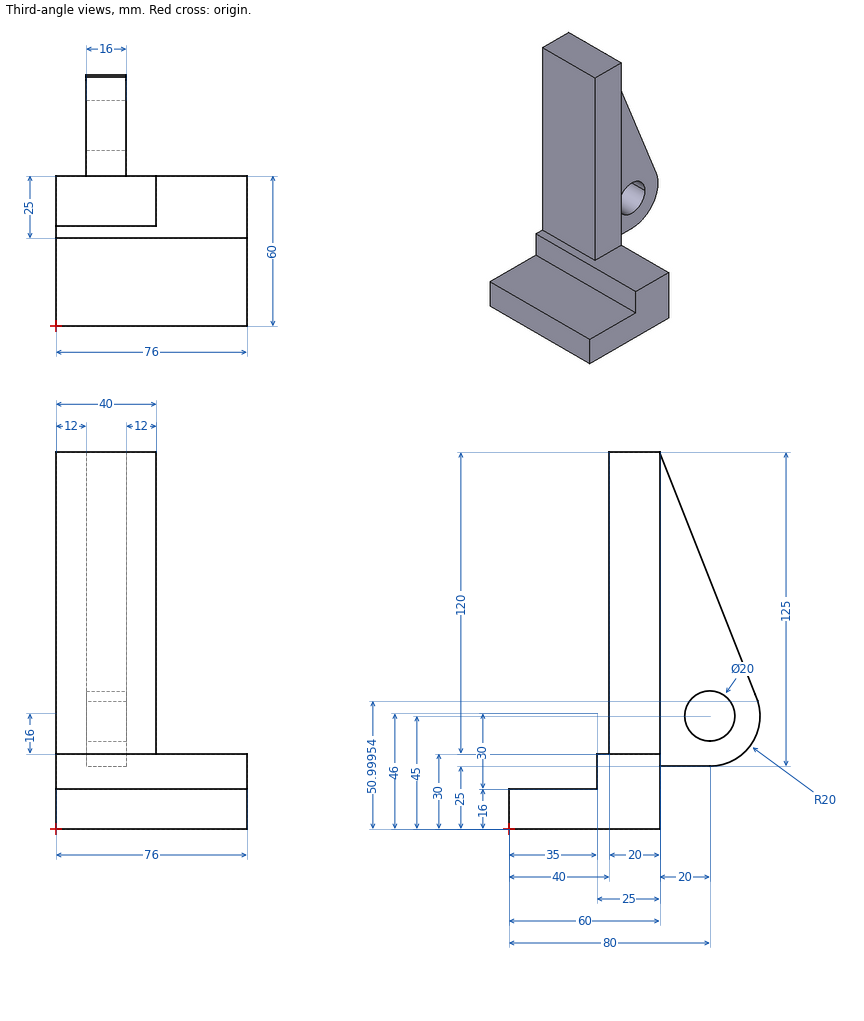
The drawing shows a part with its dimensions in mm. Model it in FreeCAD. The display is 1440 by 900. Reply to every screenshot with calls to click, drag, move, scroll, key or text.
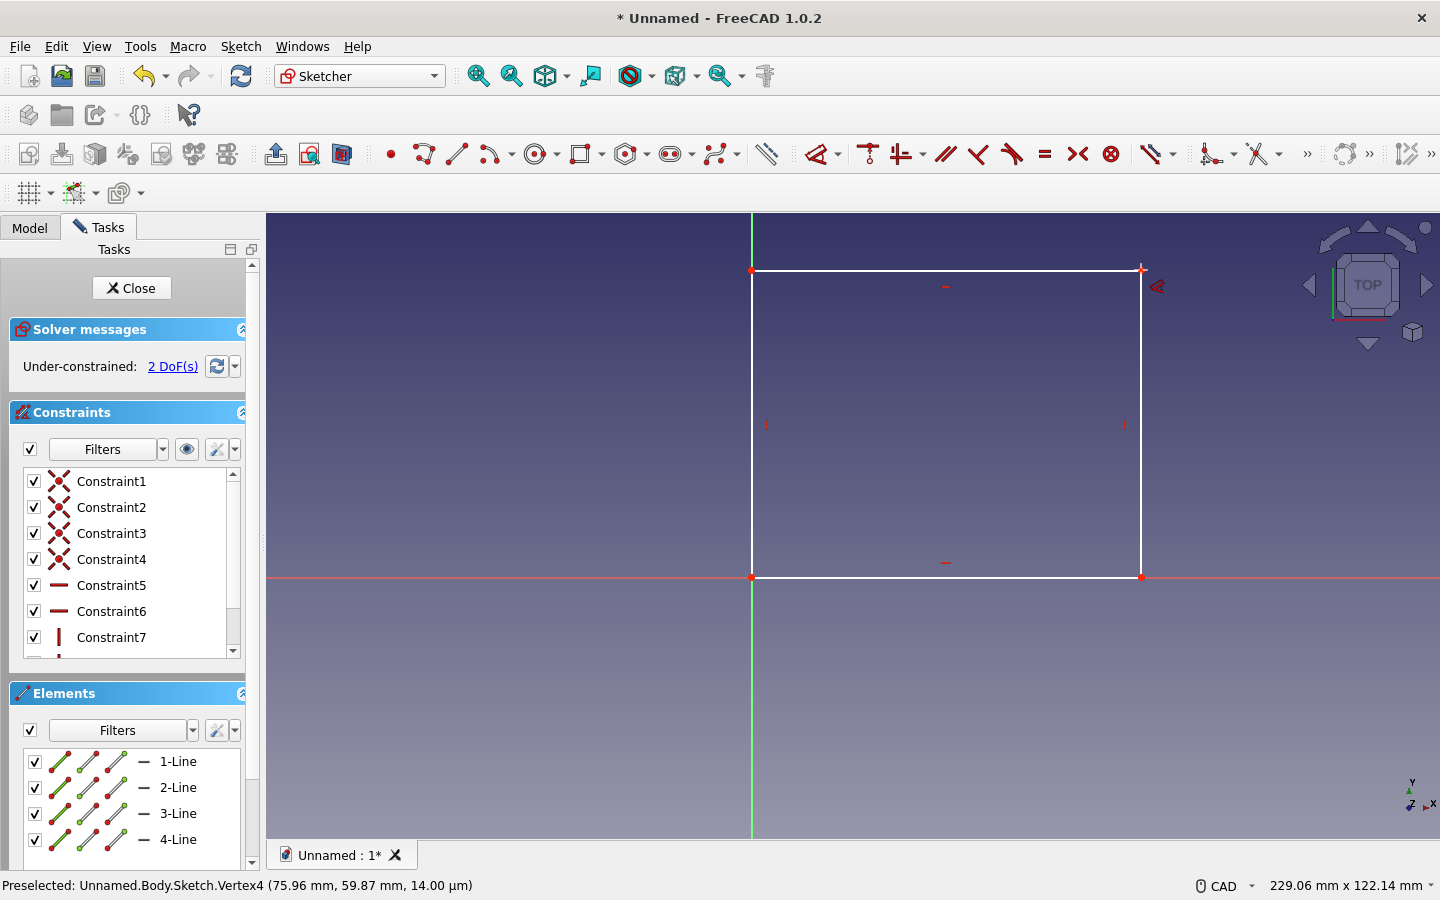
click(868, 578)
click(946, 612)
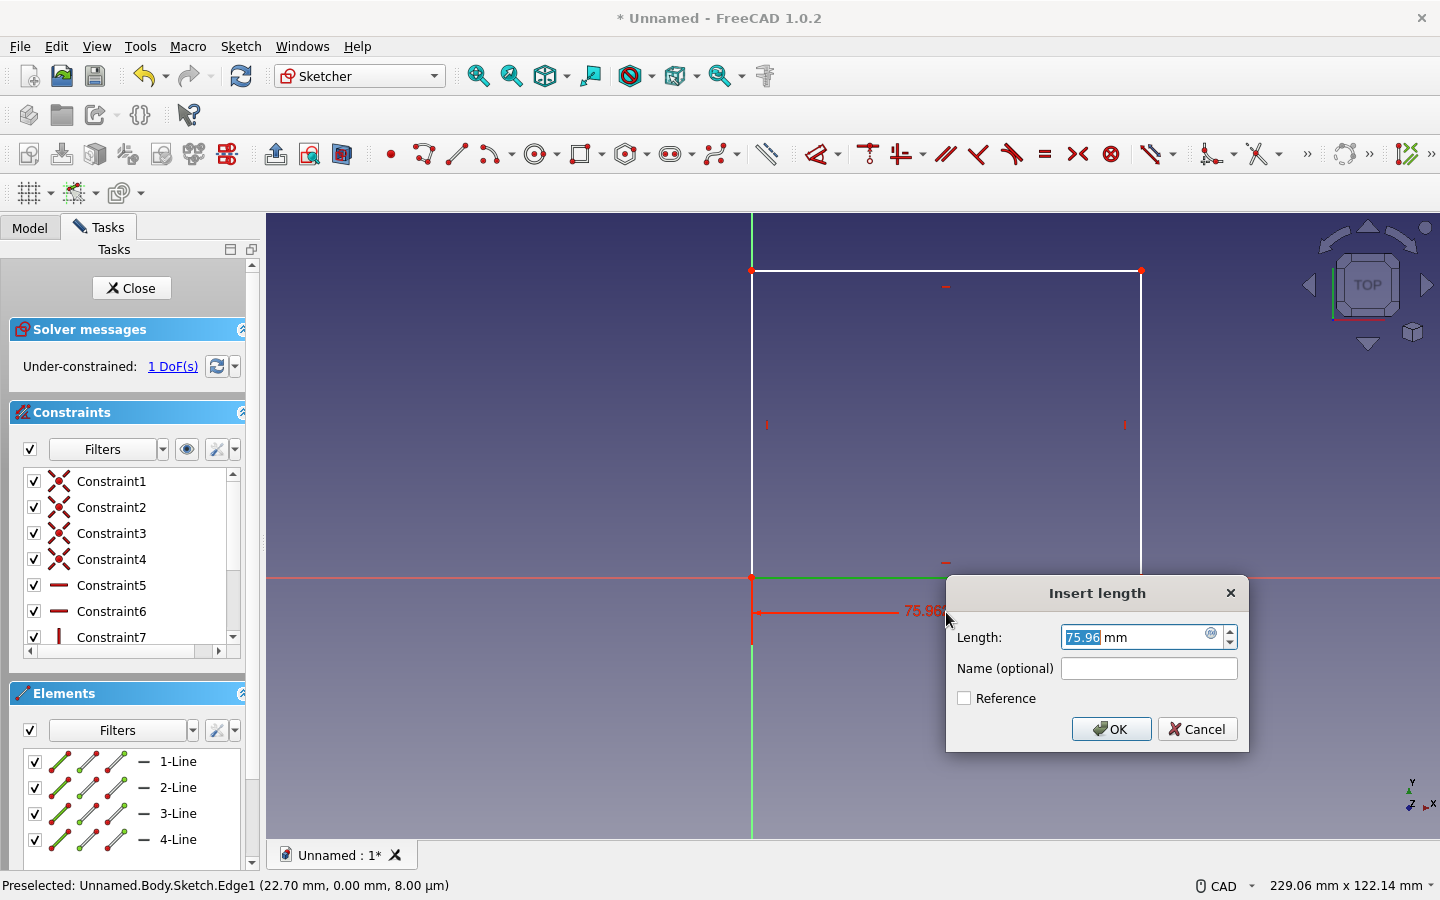
text(76)
key(Return)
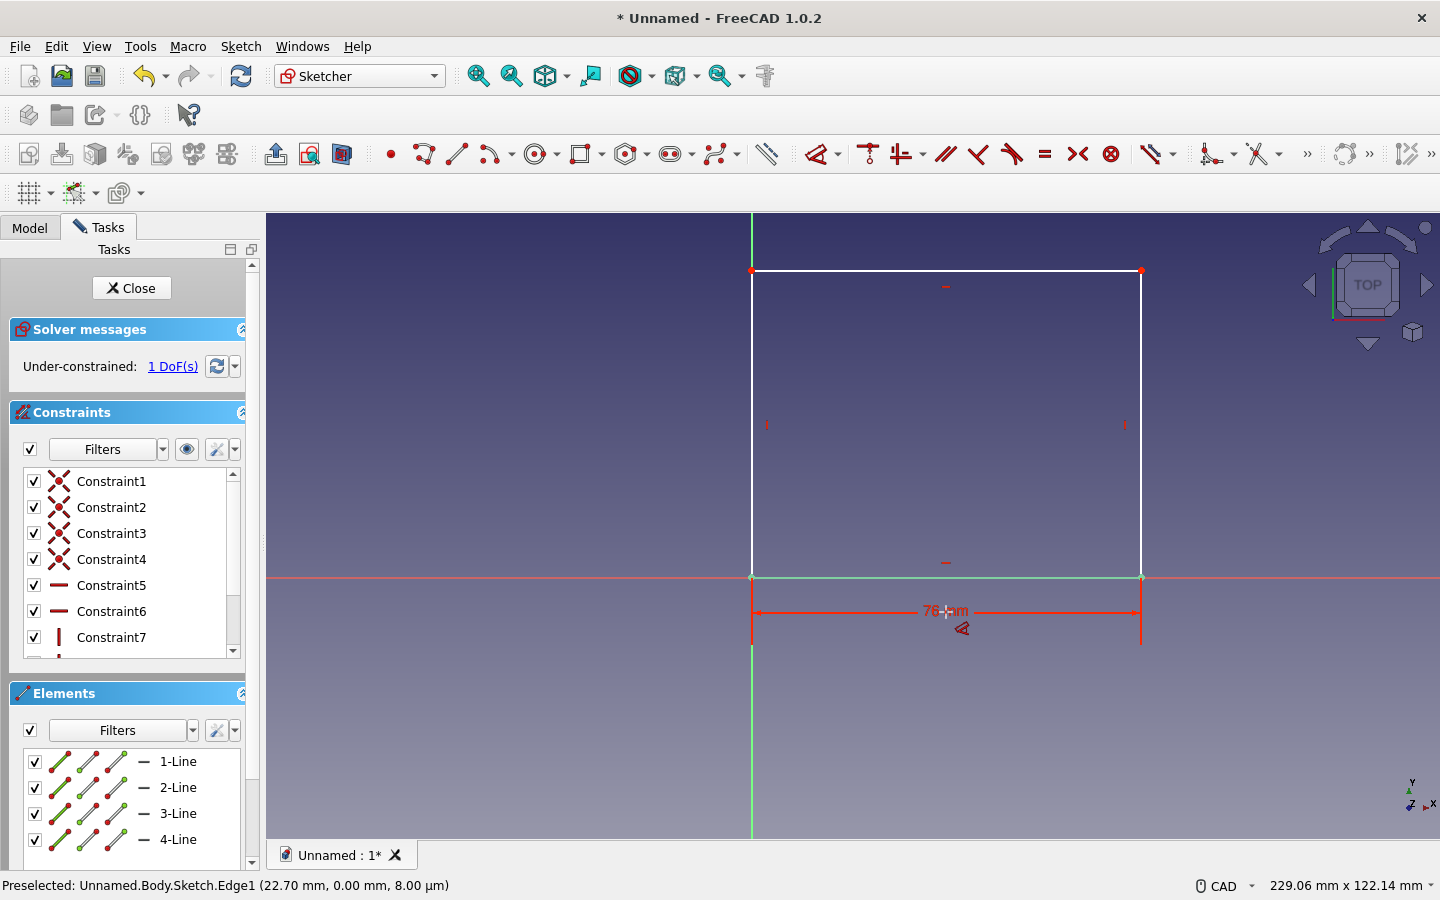
click(1141, 486)
click(1175, 424)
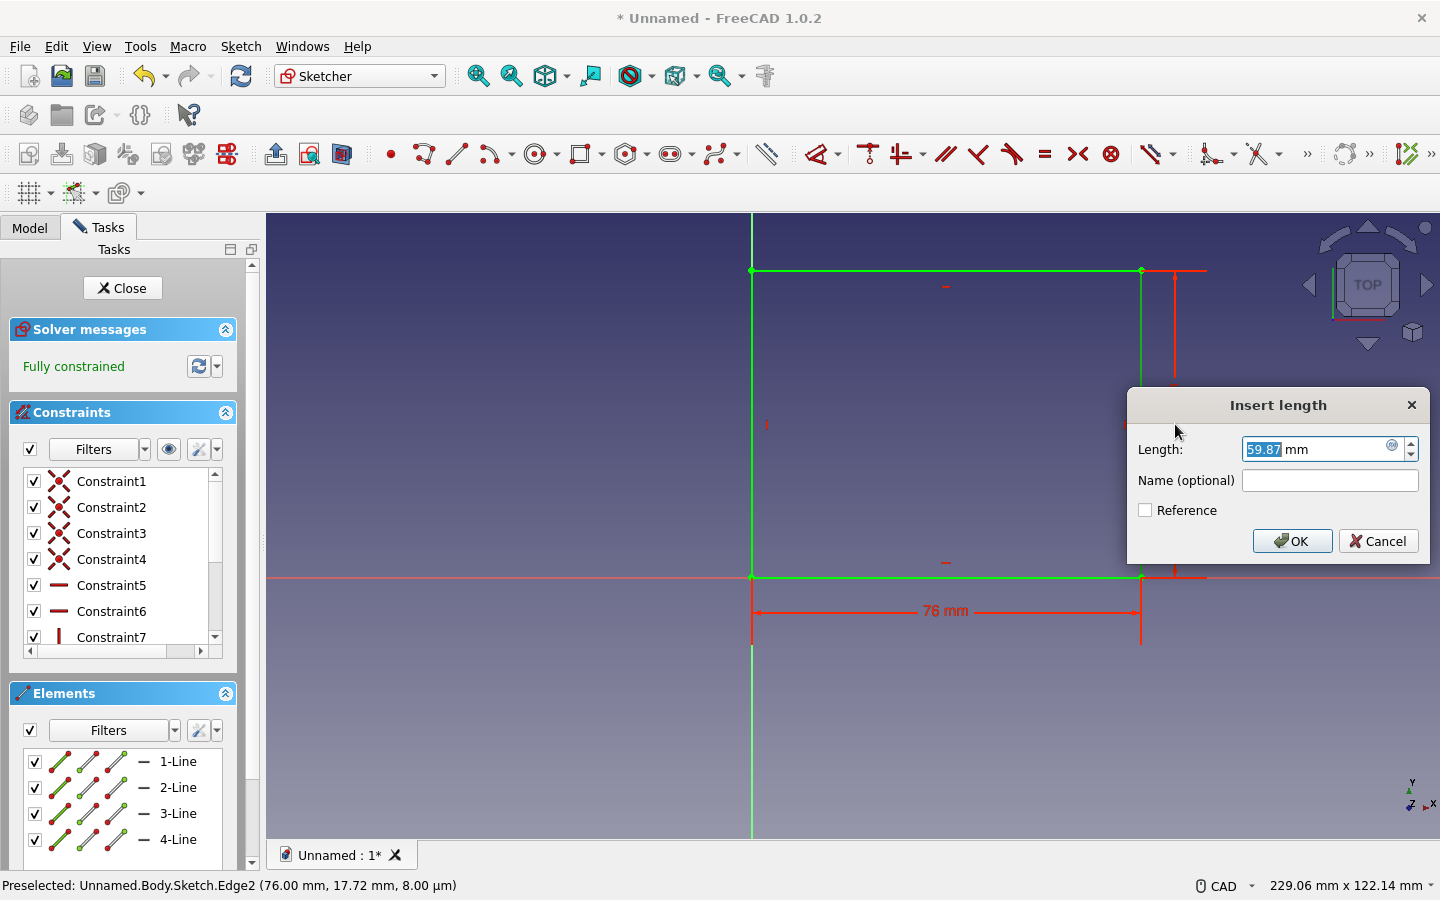
text(60)
key(Return)
key(Escape)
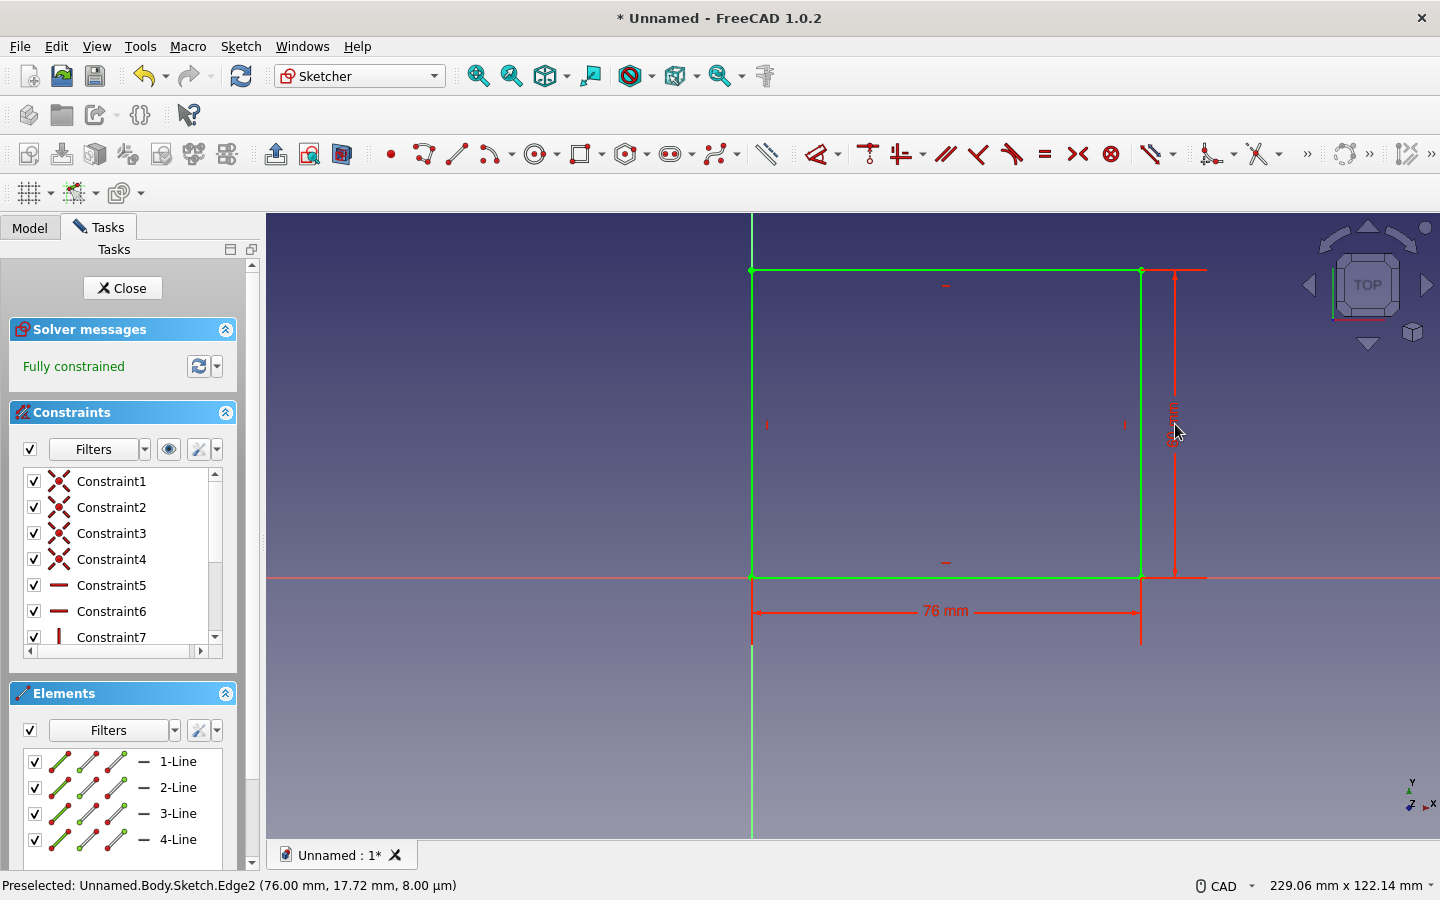
click(123, 288)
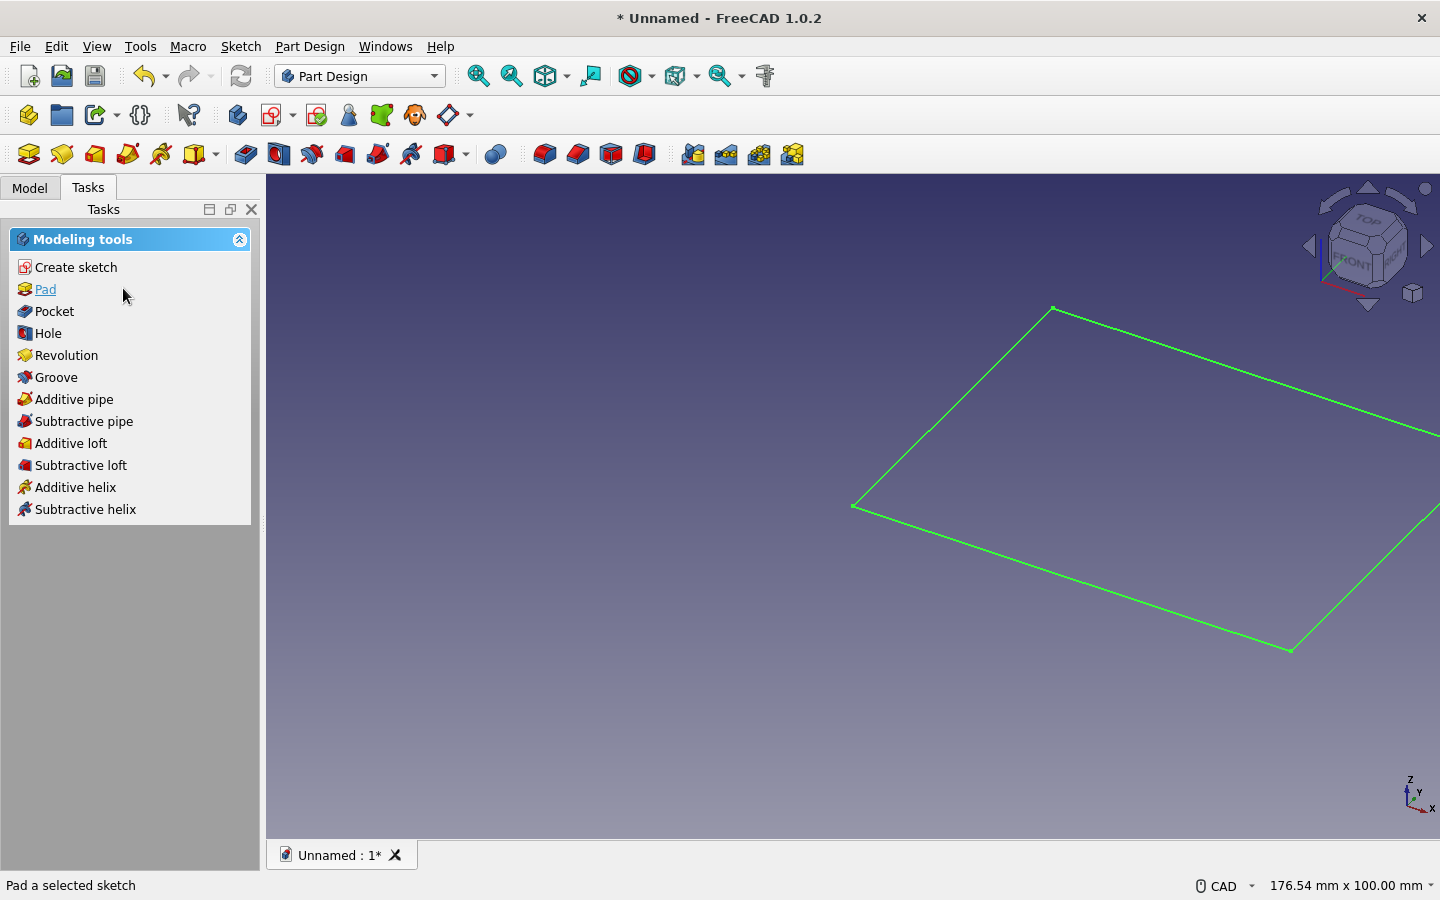
click(29, 154)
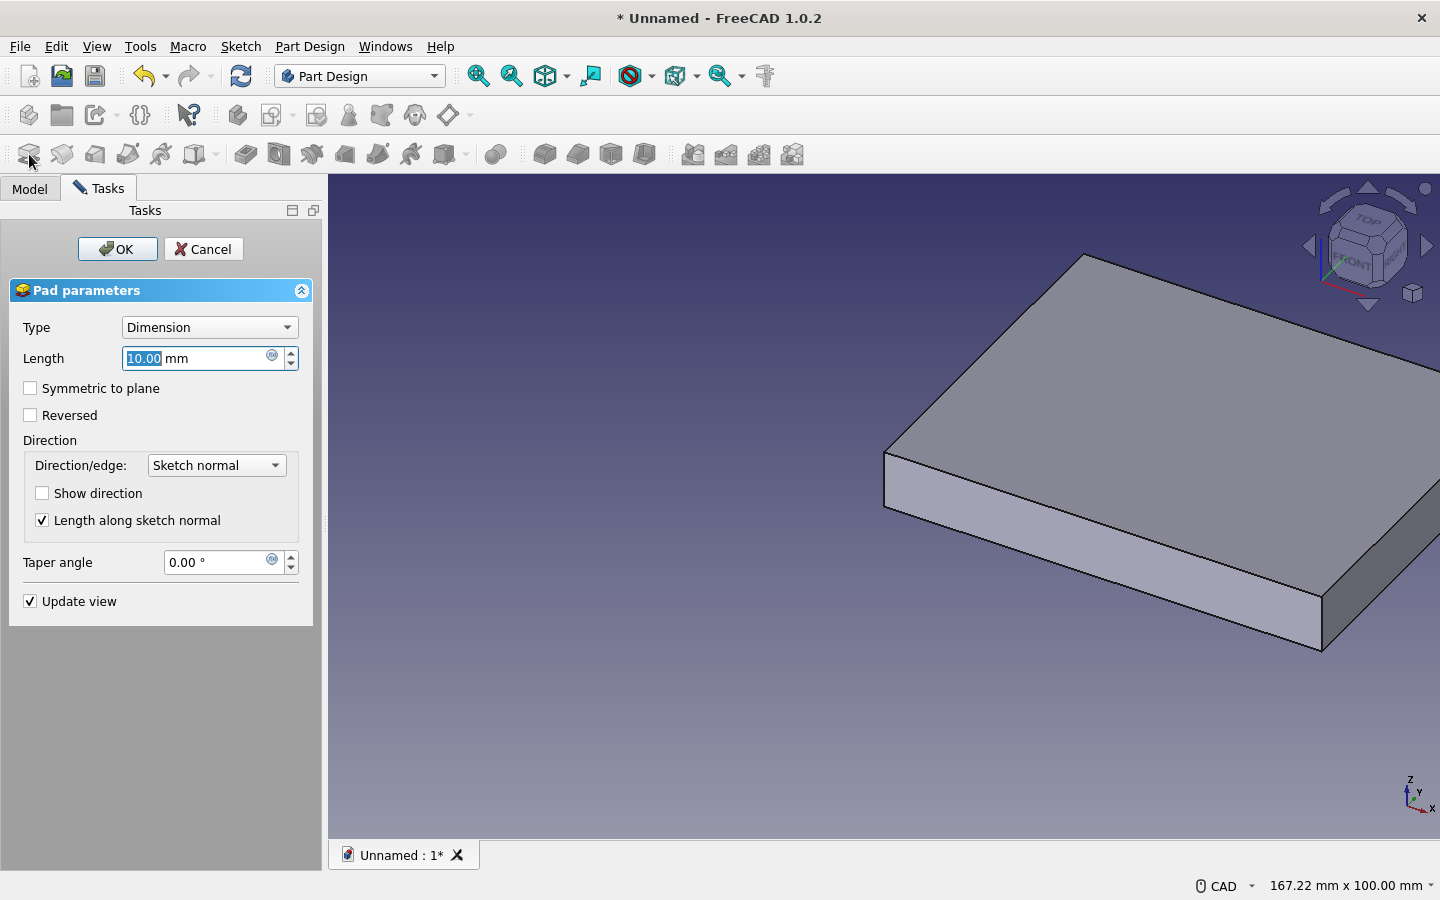
text(16)
key(Tab)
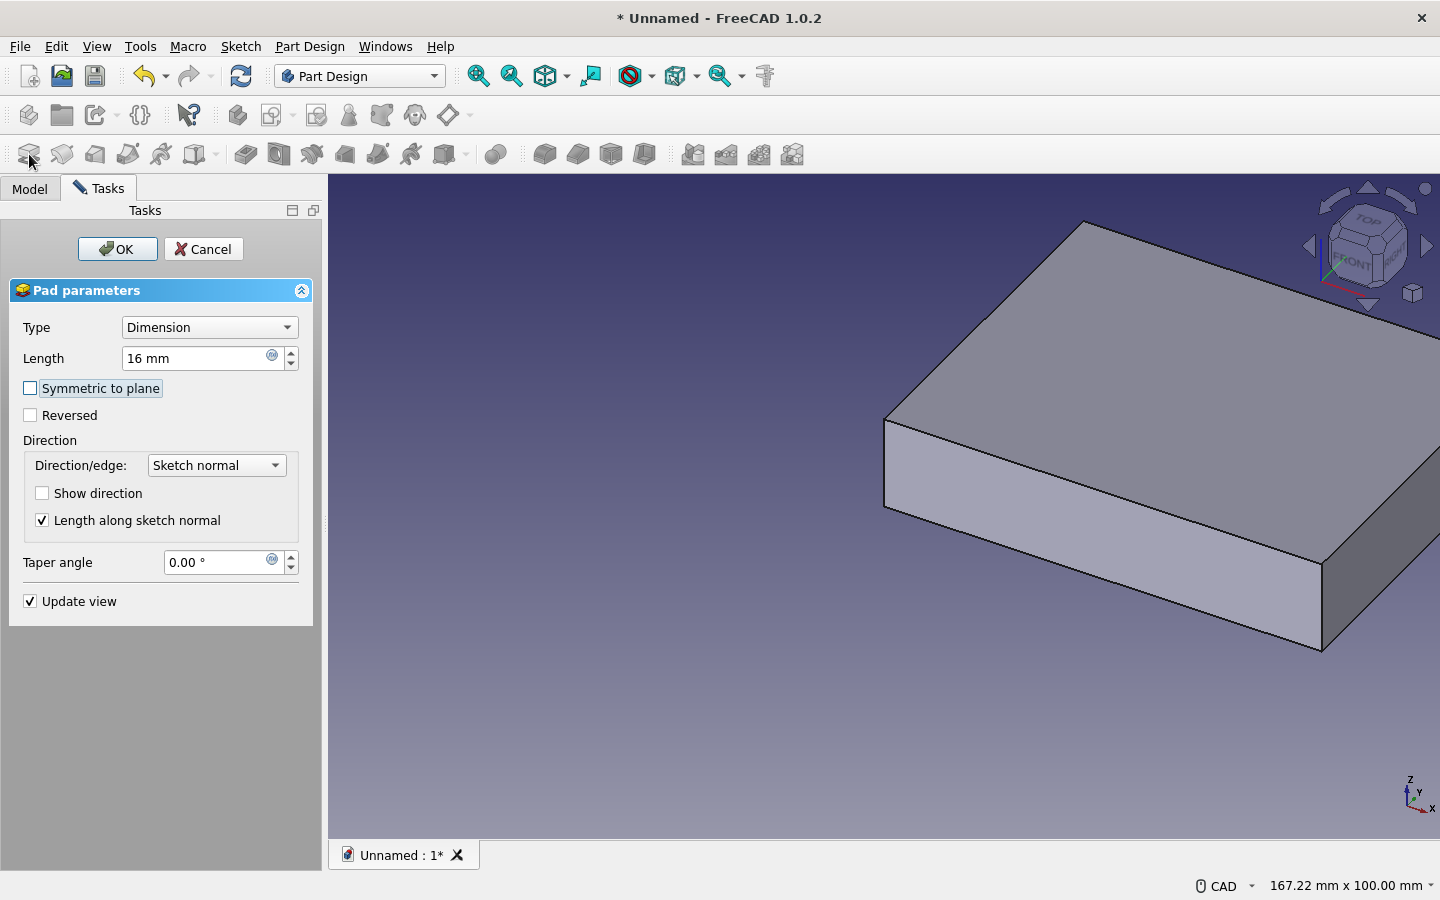
click(118, 249)